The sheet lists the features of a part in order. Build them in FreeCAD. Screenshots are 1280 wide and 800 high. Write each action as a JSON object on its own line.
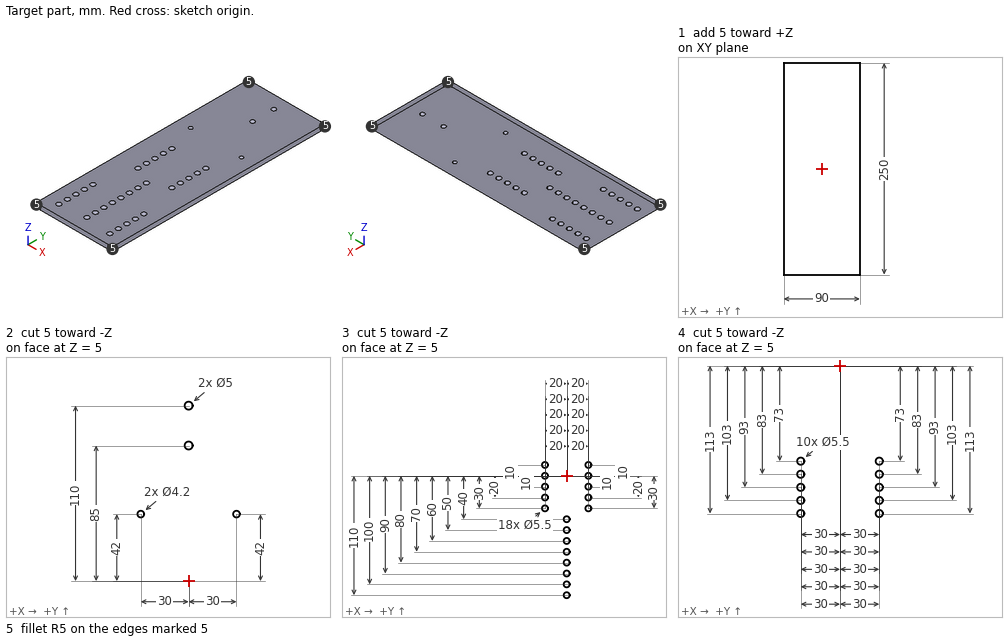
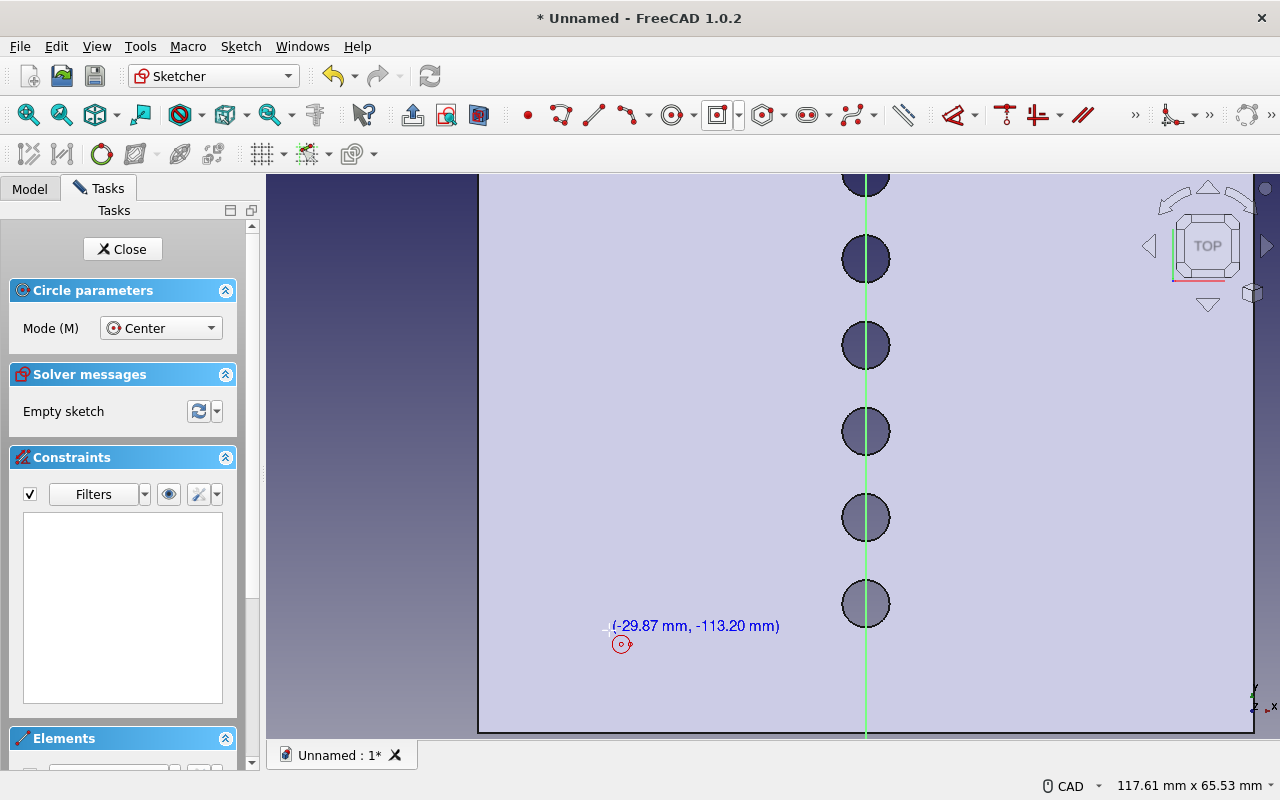
{"action": "left_click", "coordinate": [607, 630]}
{"action": "mouse_move", "coordinate": [624, 613]}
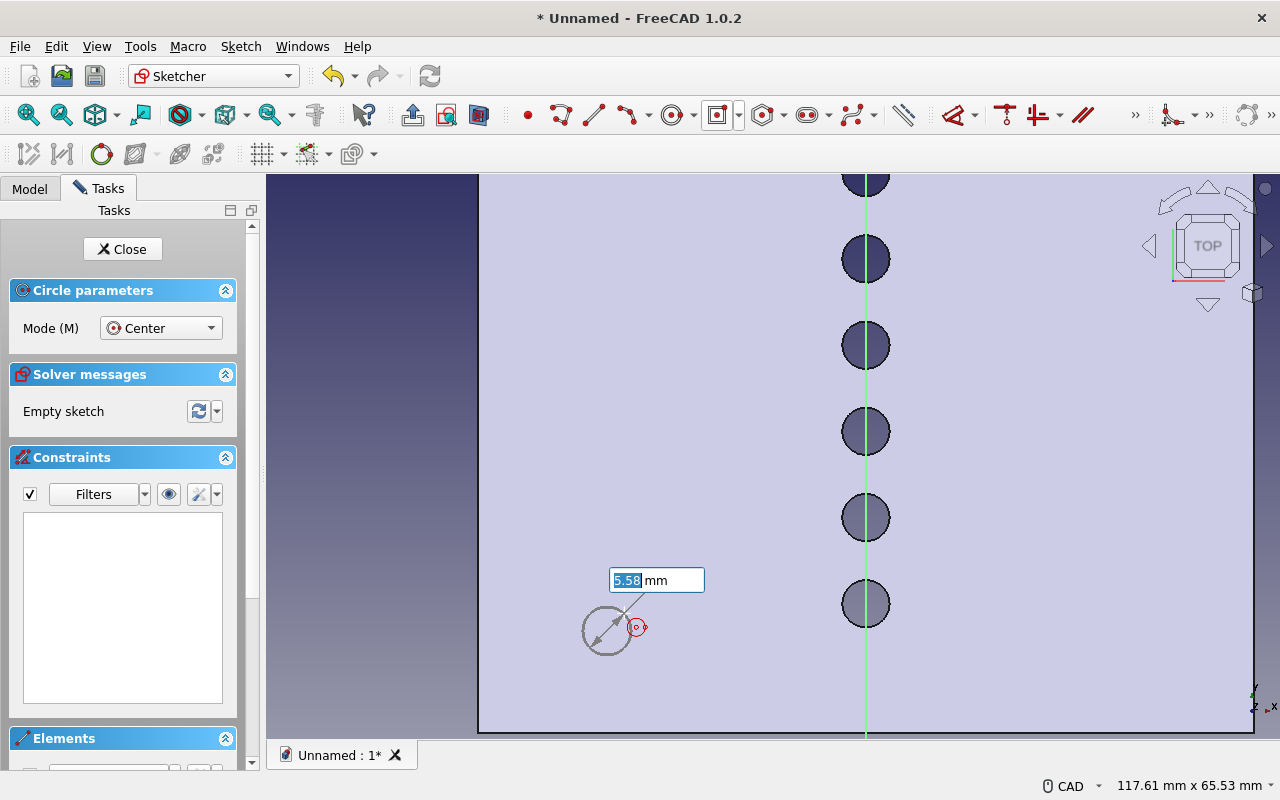
{"action": "type", "text": "5.5"}
{"action": "key", "text": "Return"}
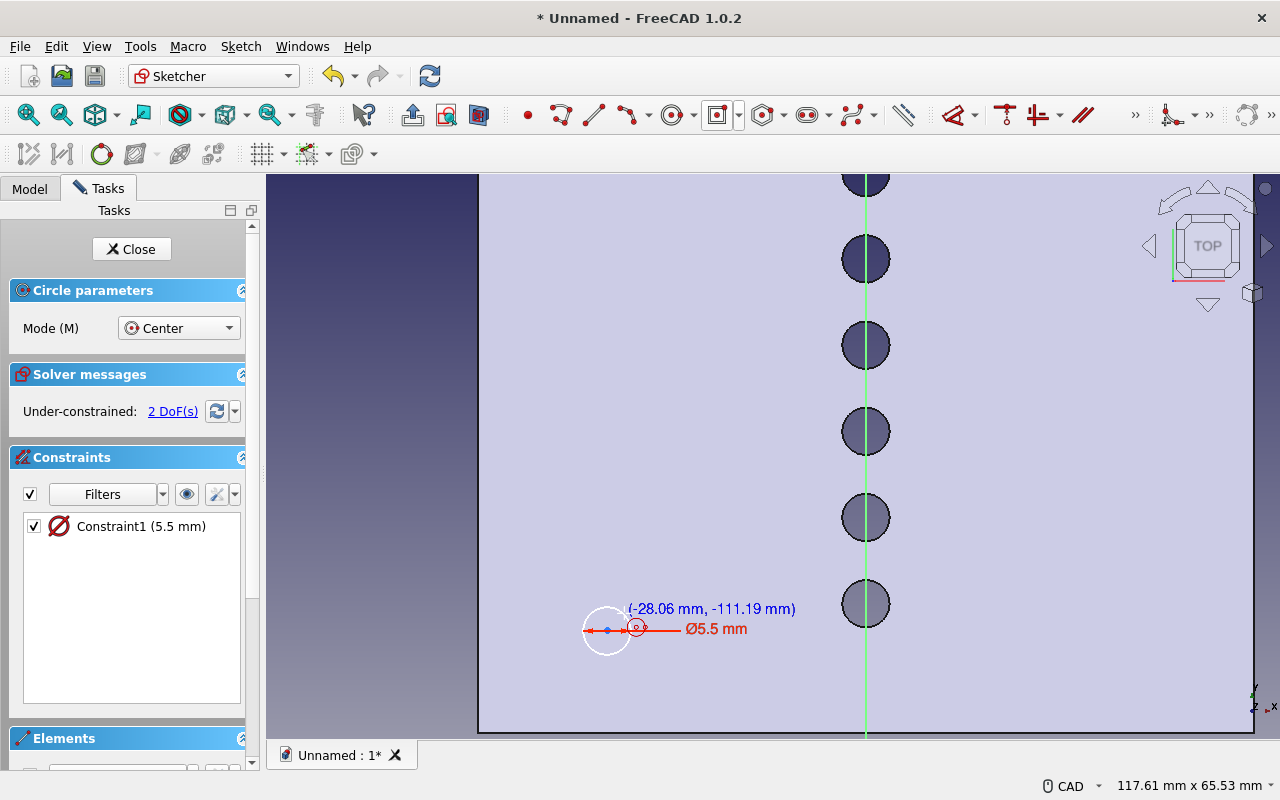
{"action": "scroll", "coordinate": [611, 632], "scroll_direction": "down", "scroll_amount": 5}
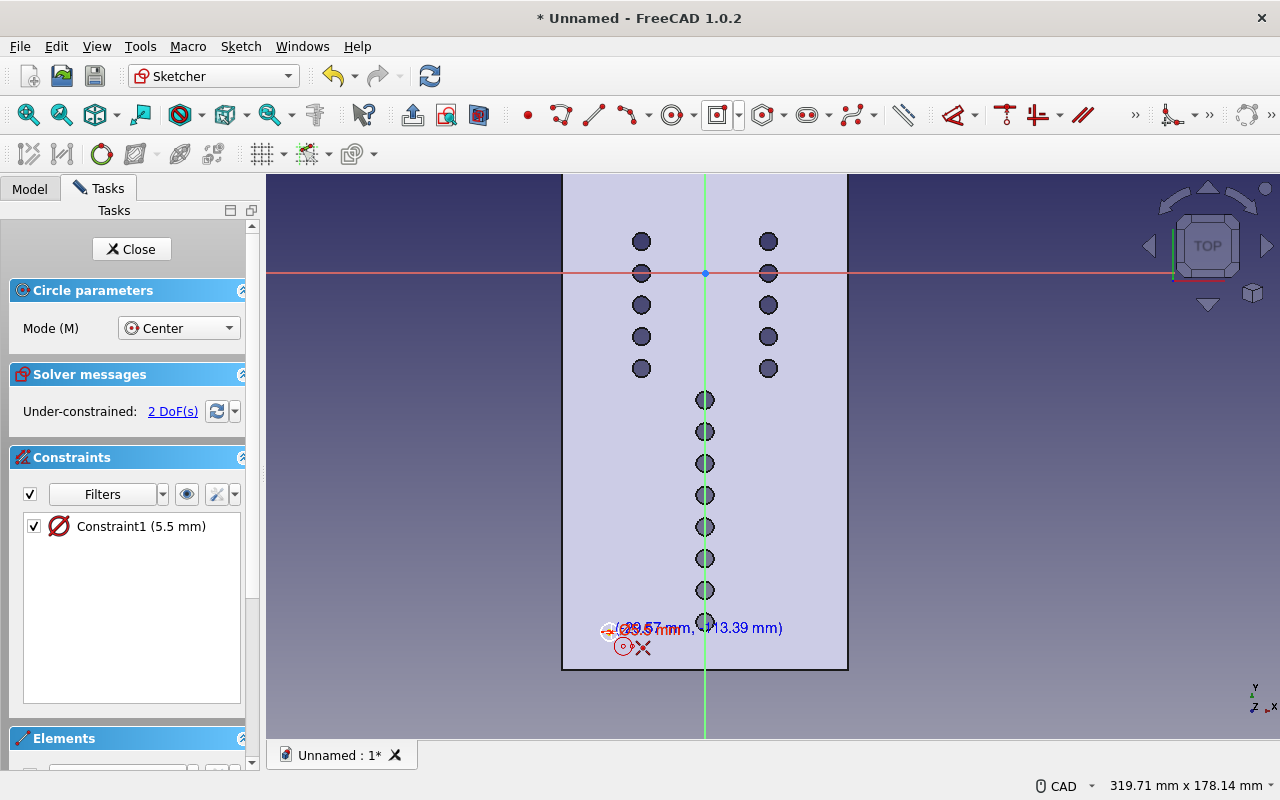
{"action": "scroll", "coordinate": [800, 632], "scroll_direction": "up", "scroll_amount": 5}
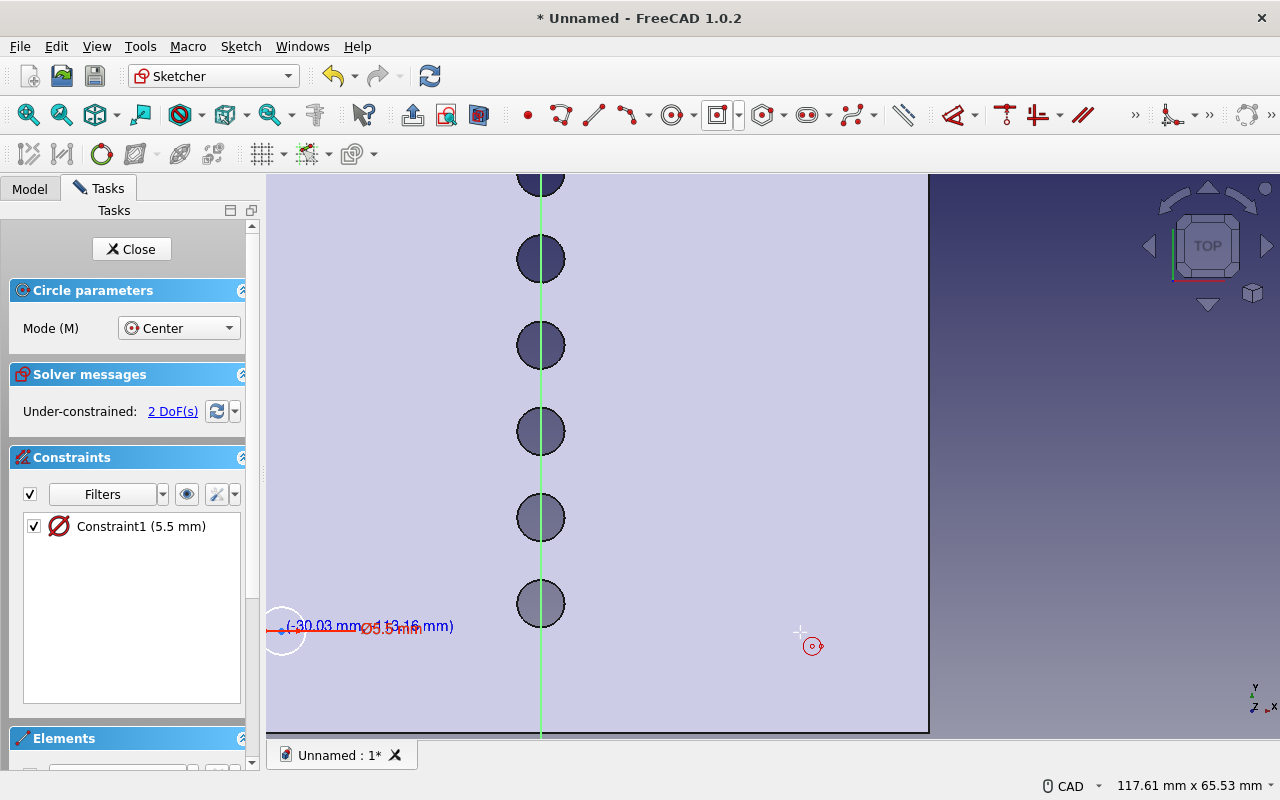
{"action": "left_click", "coordinate": [800, 630]}
{"action": "mouse_move", "coordinate": [816, 613]}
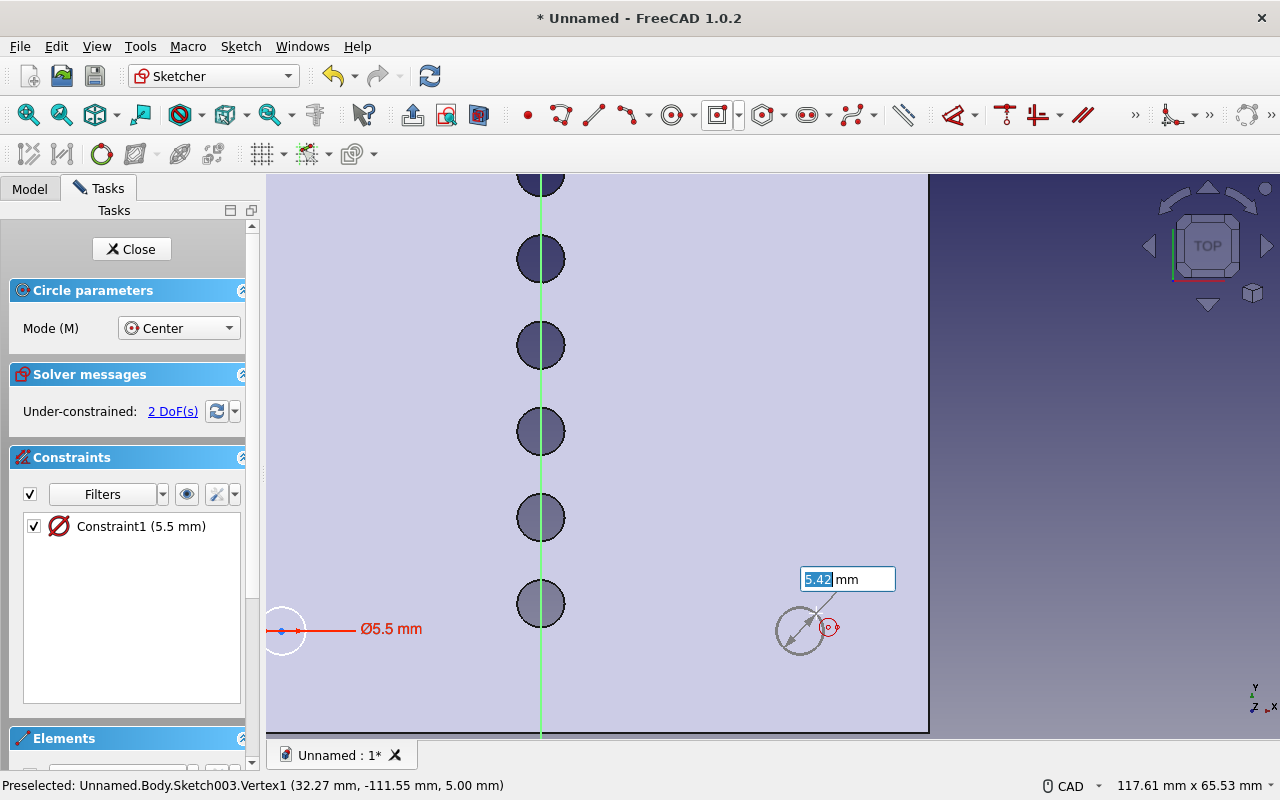
{"action": "type", "text": "5.5"}
{"action": "key", "text": "Return"}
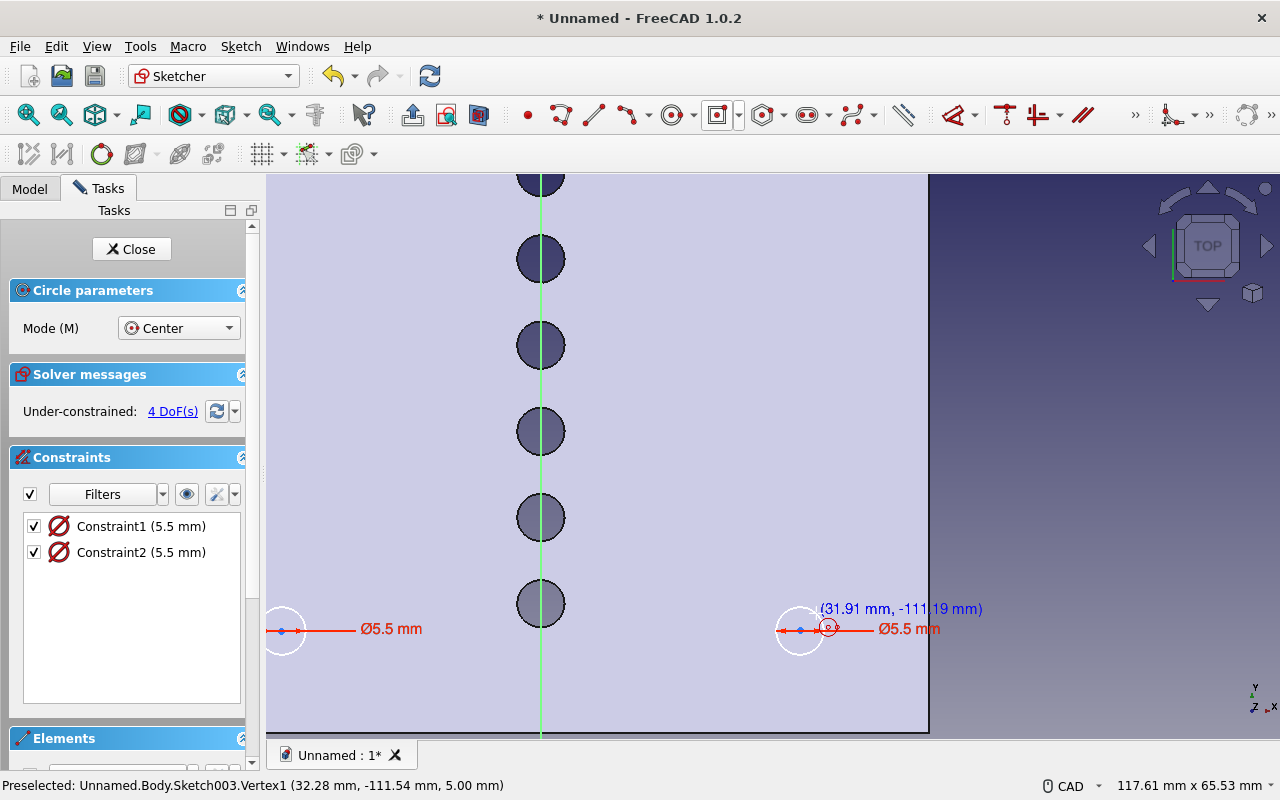
{"action": "scroll", "coordinate": [800, 632], "scroll_direction": "down", "scroll_amount": 5}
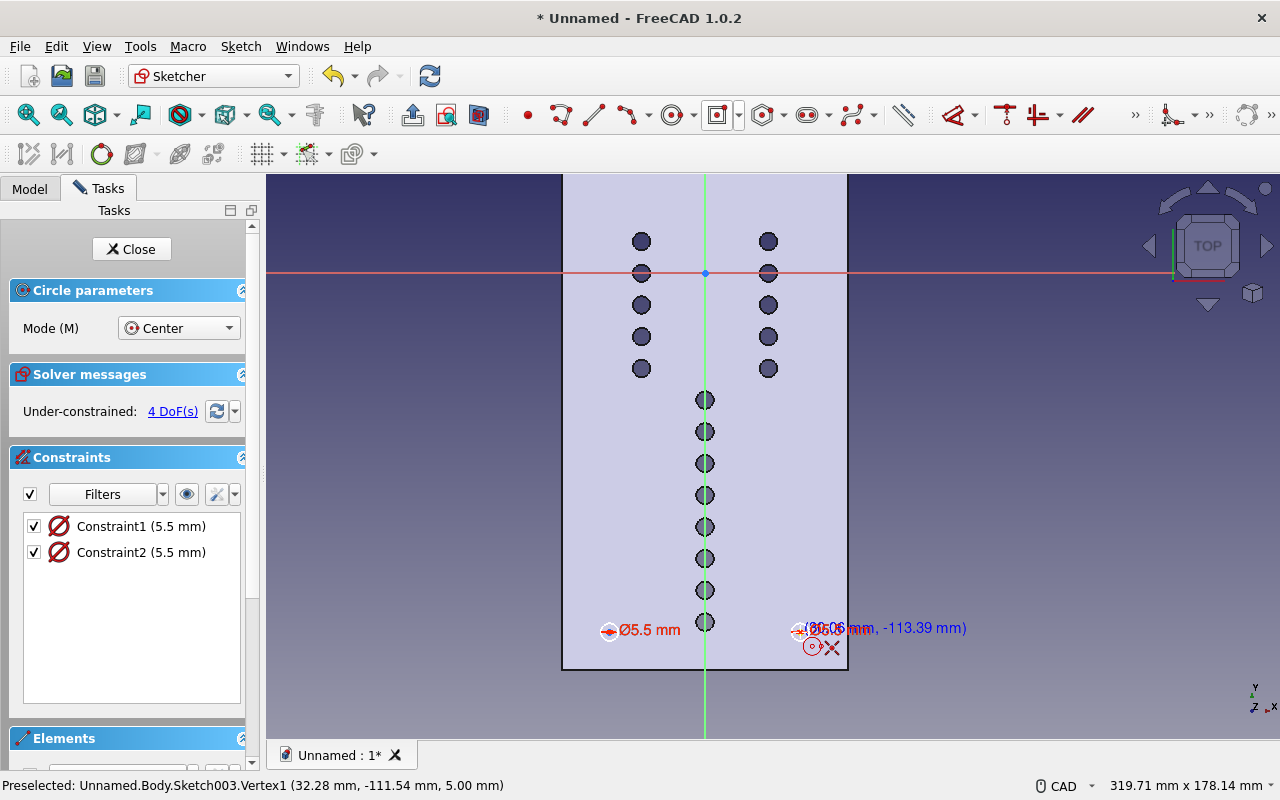
{"action": "scroll", "coordinate": [610, 600], "scroll_direction": "up", "scroll_amount": 5}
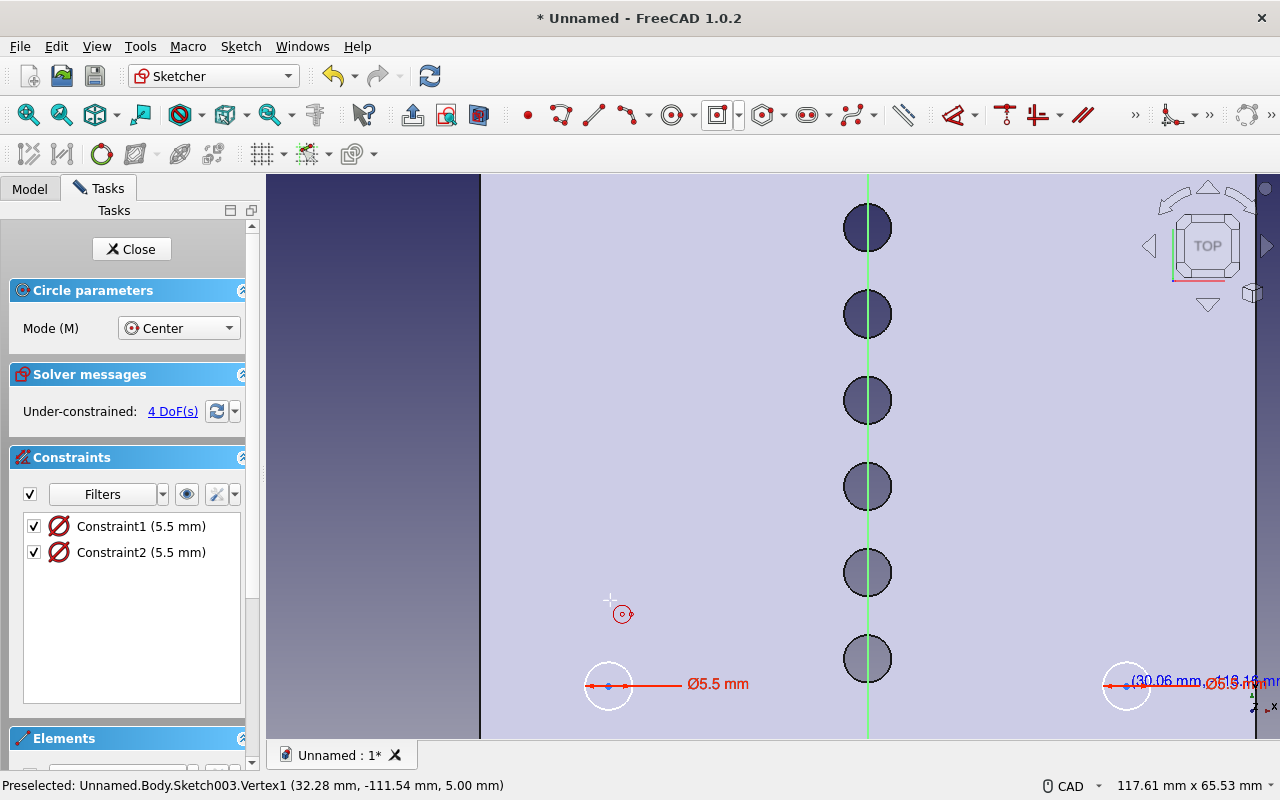
{"action": "left_click", "coordinate": [609, 599]}
{"action": "mouse_move", "coordinate": [626, 582]}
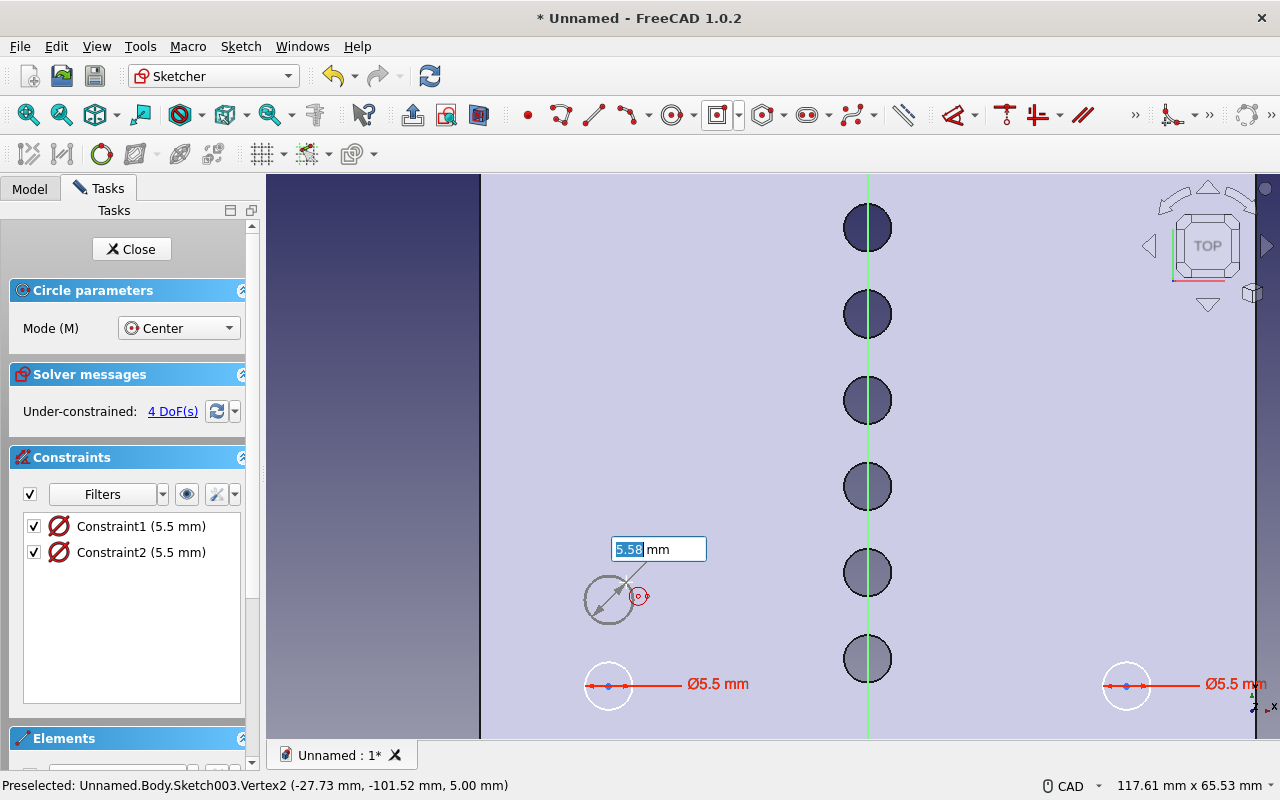
{"action": "type", "text": "5.5"}
{"action": "key", "text": "Return"}